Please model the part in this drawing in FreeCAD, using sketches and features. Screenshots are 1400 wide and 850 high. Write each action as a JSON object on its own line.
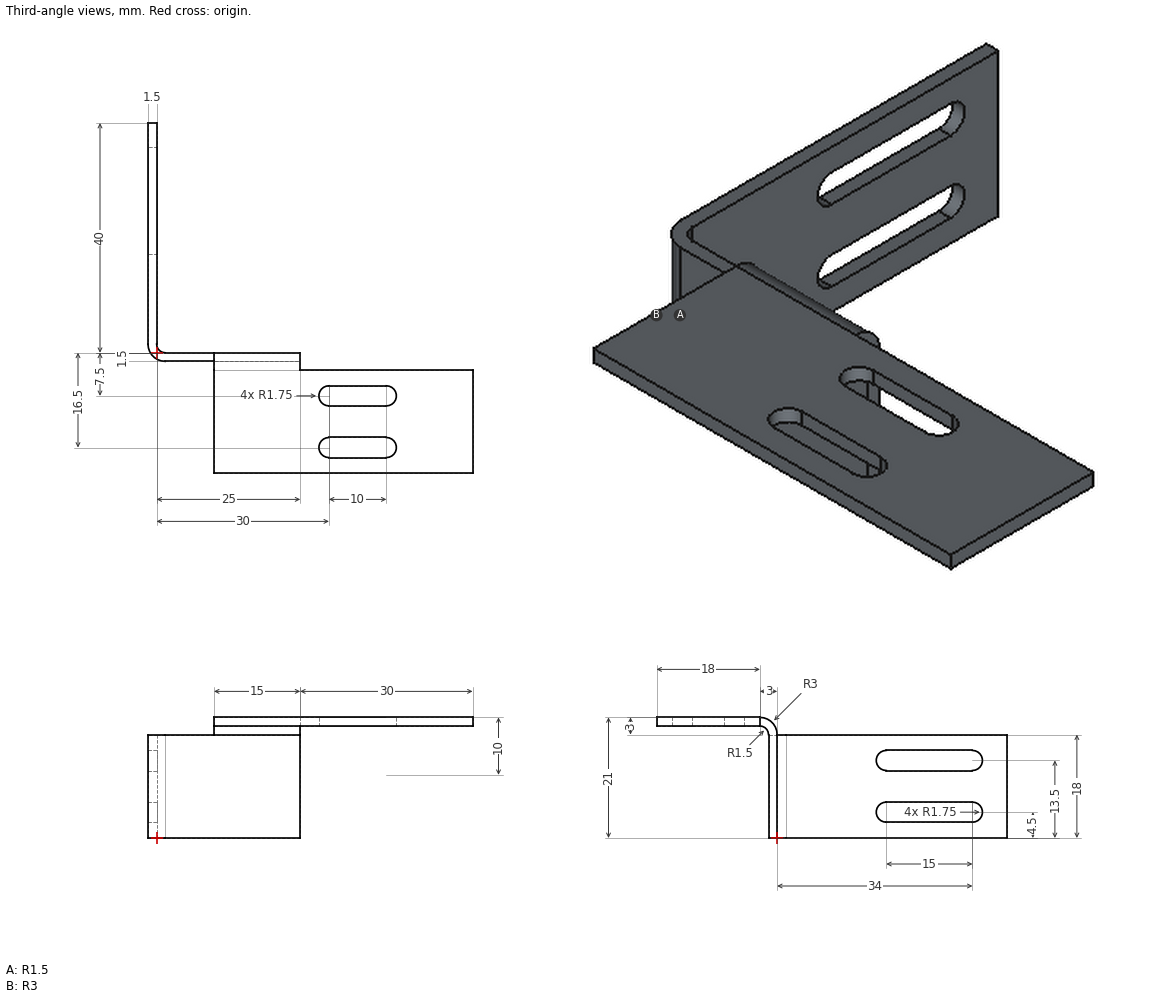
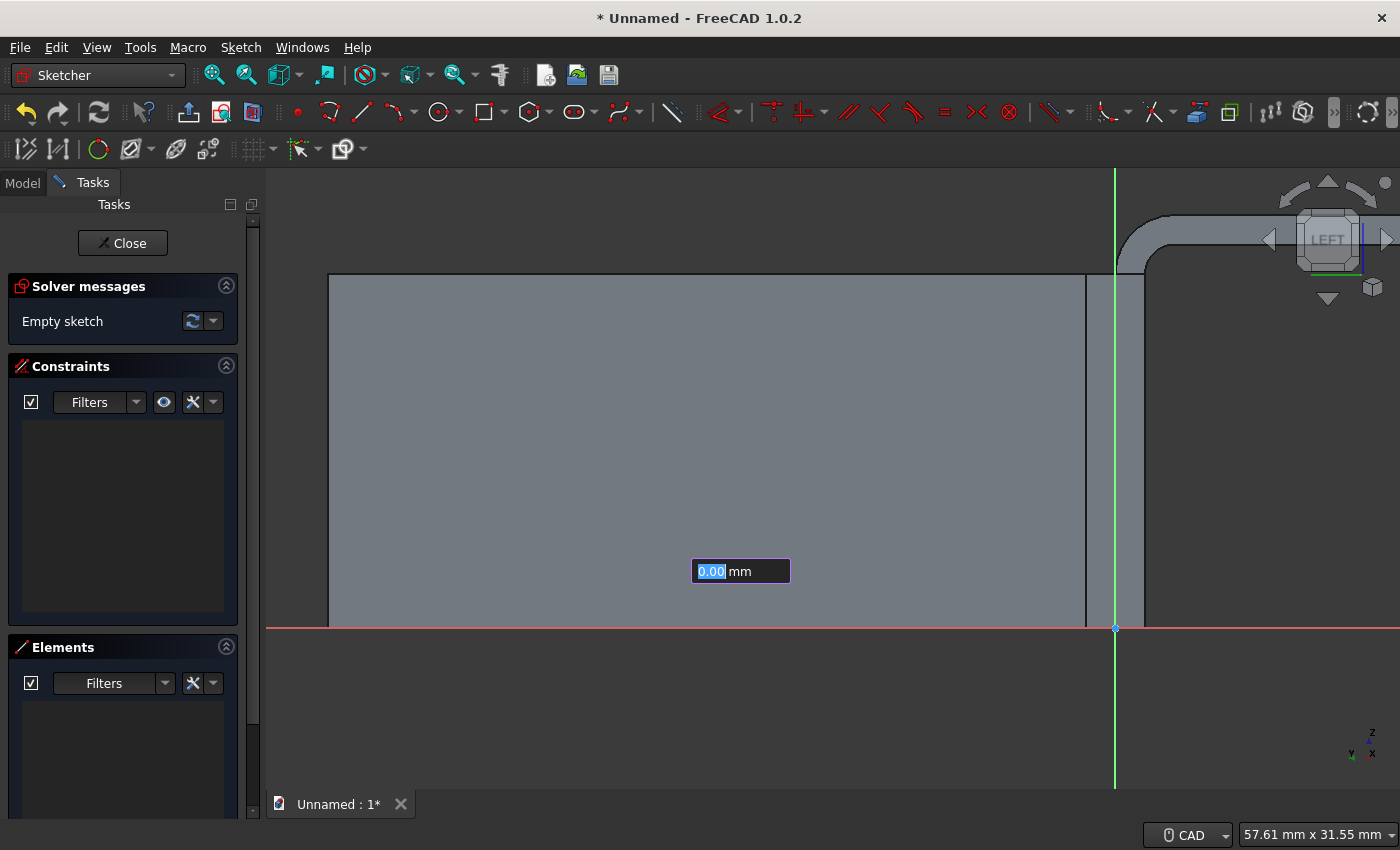
{"action": "left_click", "coordinate": [594, 505]}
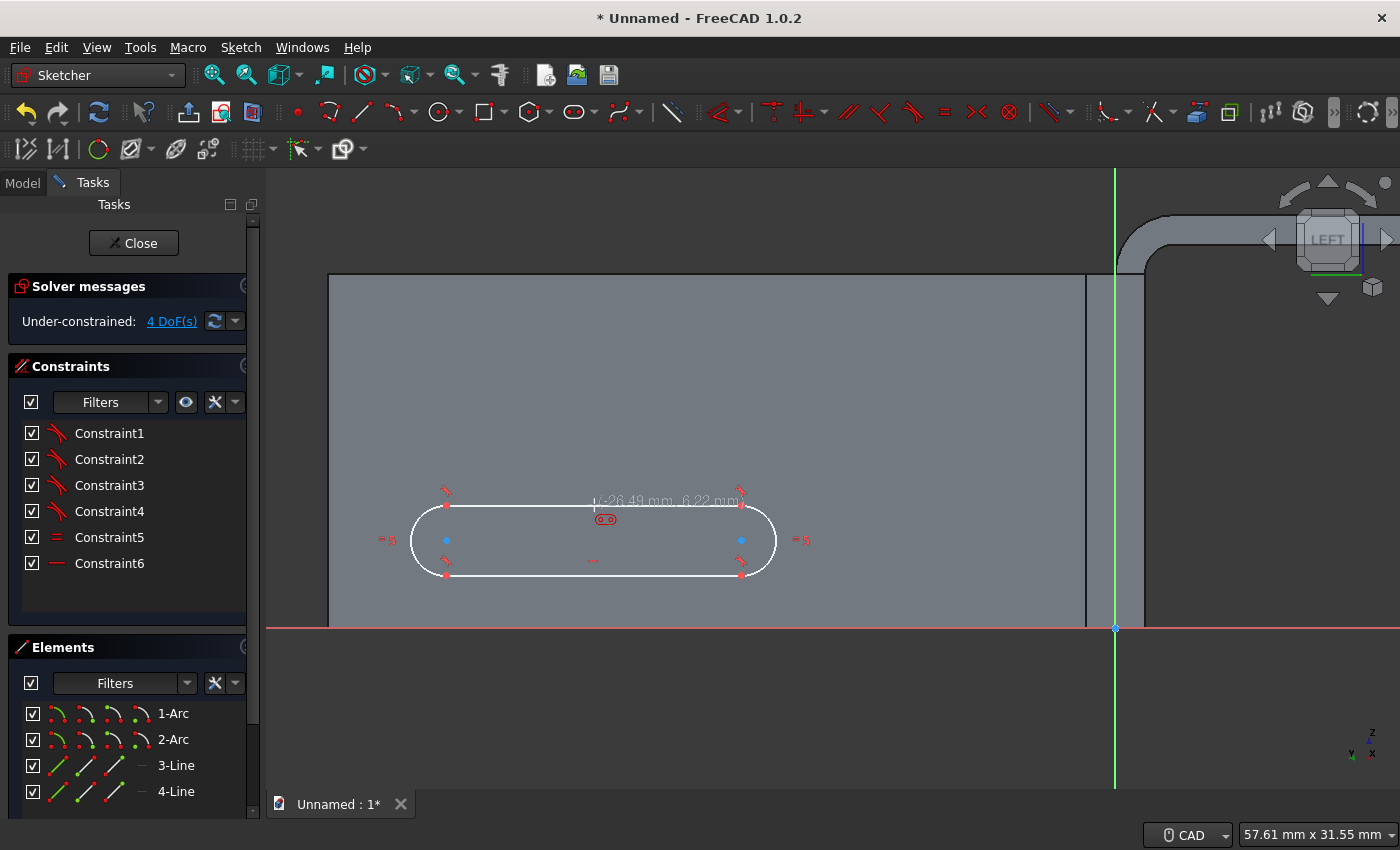
{"action": "left_click", "coordinate": [446, 363]}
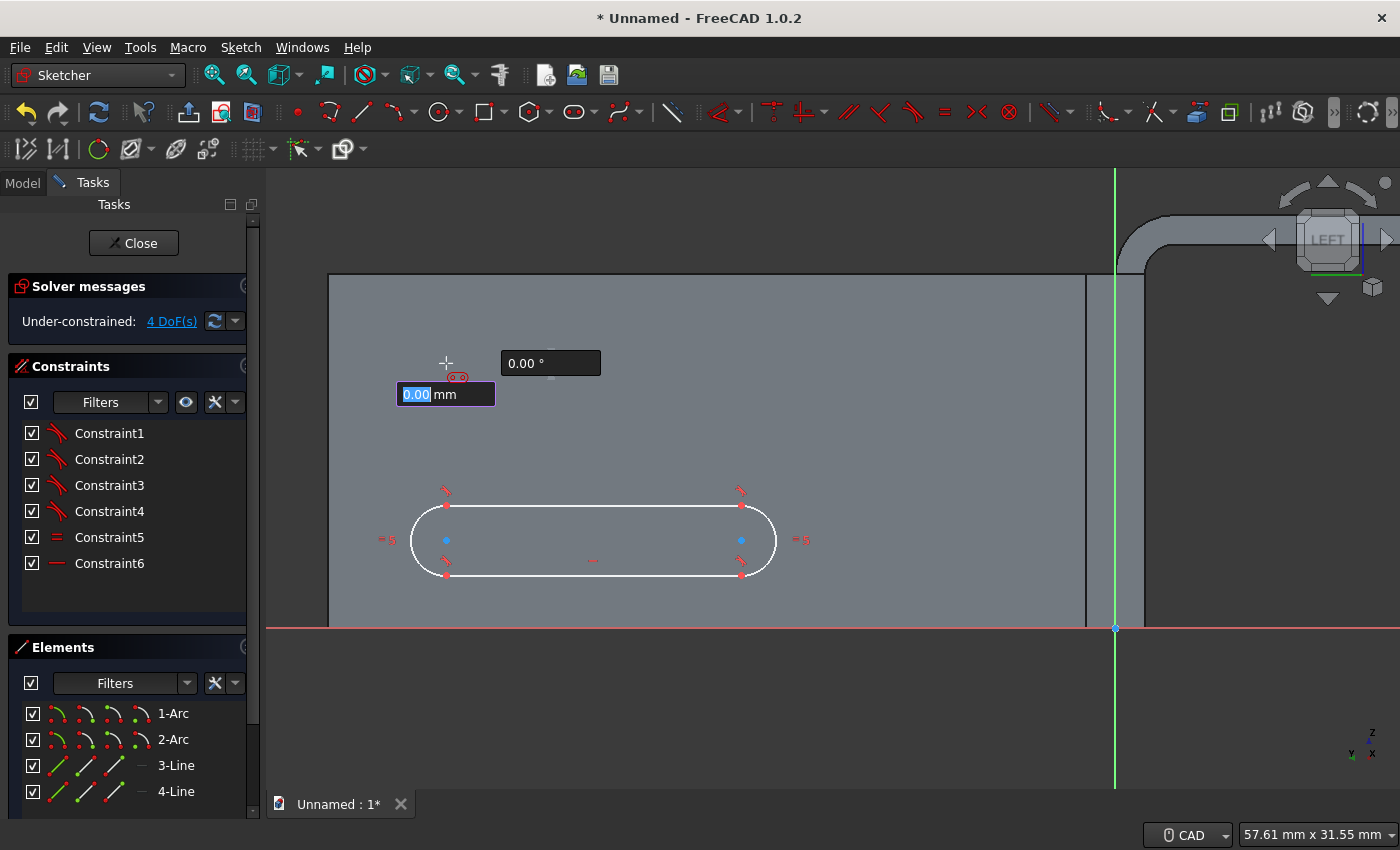
{"action": "left_click", "coordinate": [741, 363]}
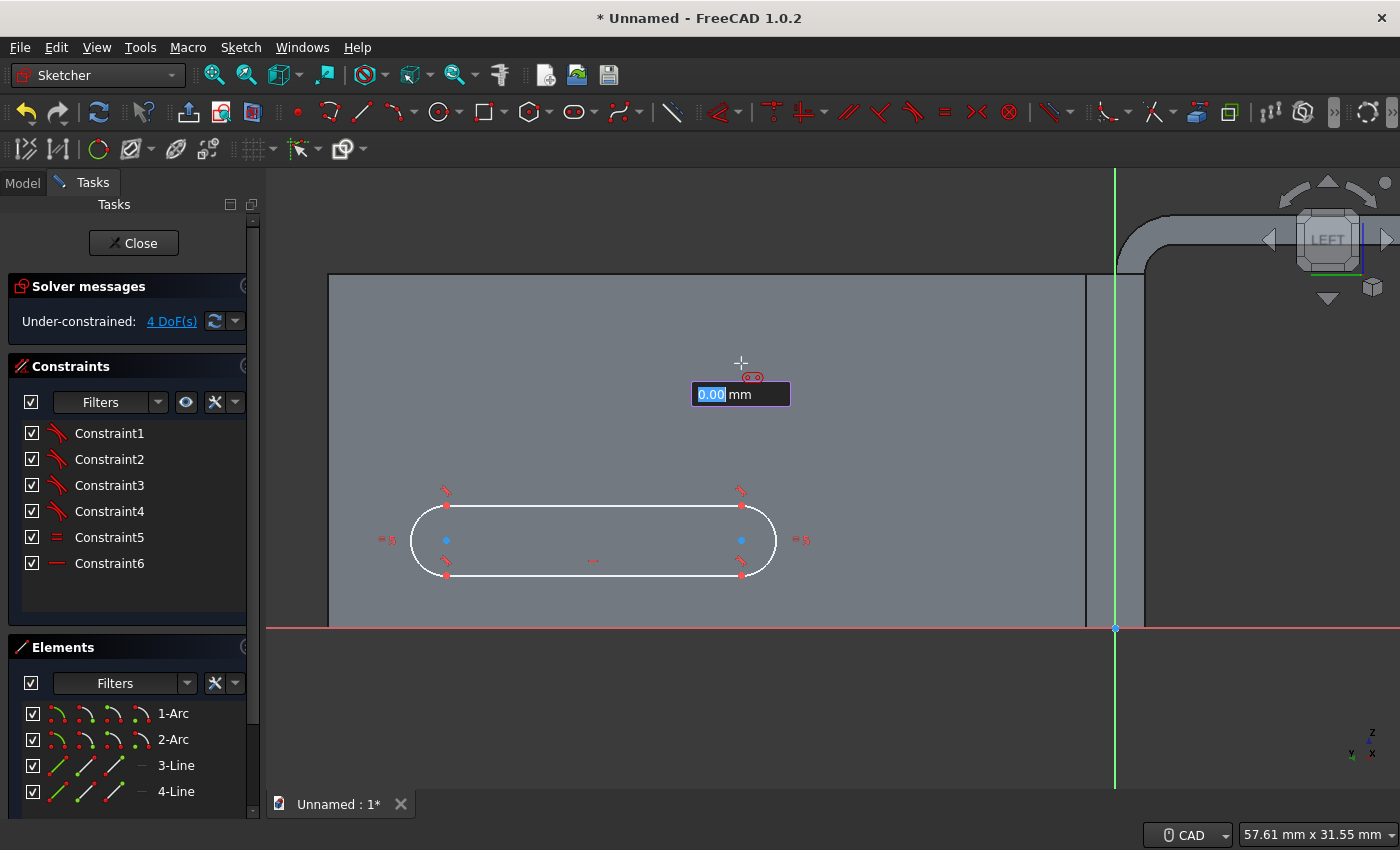
{"action": "left_click", "coordinate": [594, 397]}
{"action": "key", "text": "Escape"}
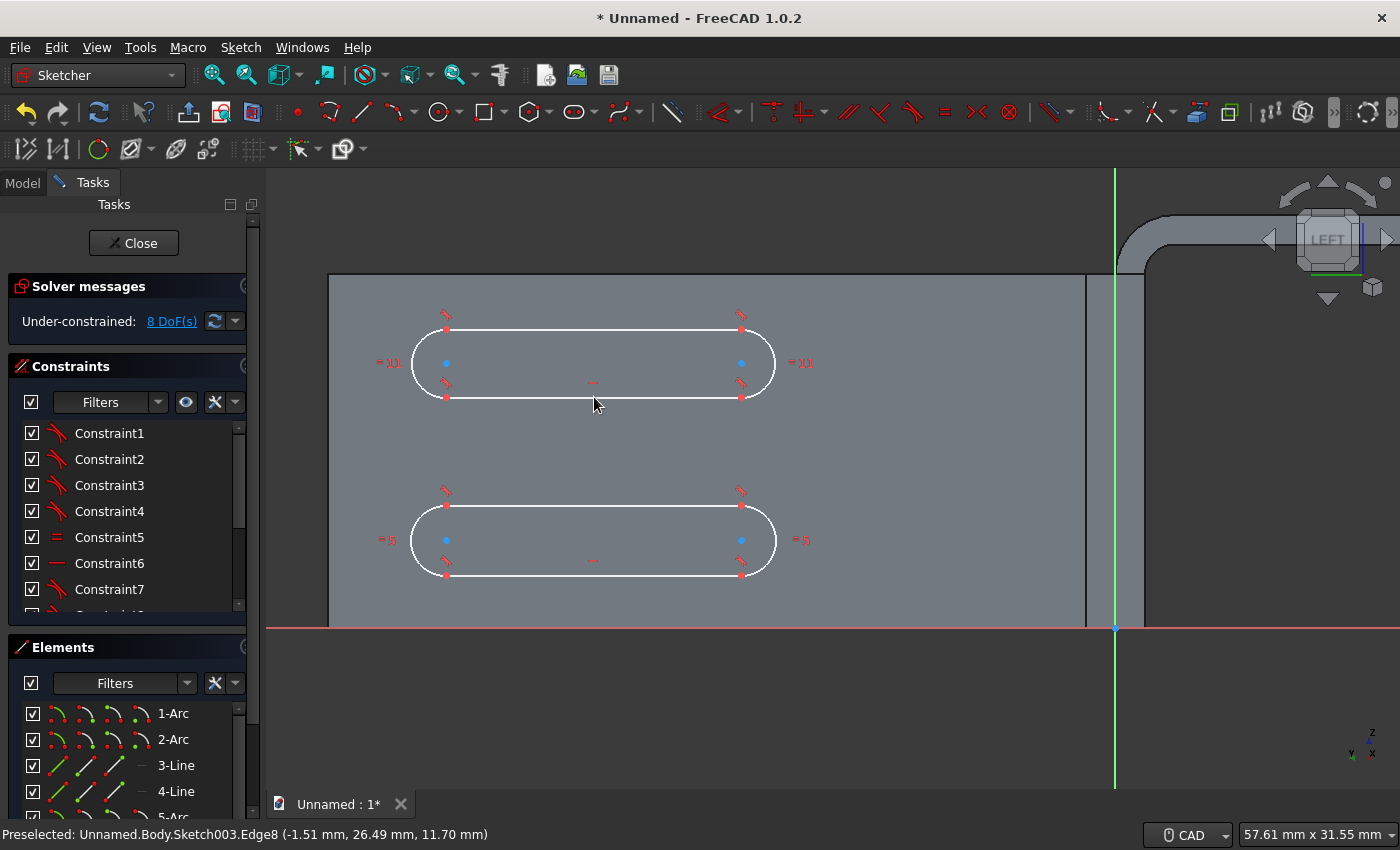
{"action": "left_click", "coordinate": [418, 520]}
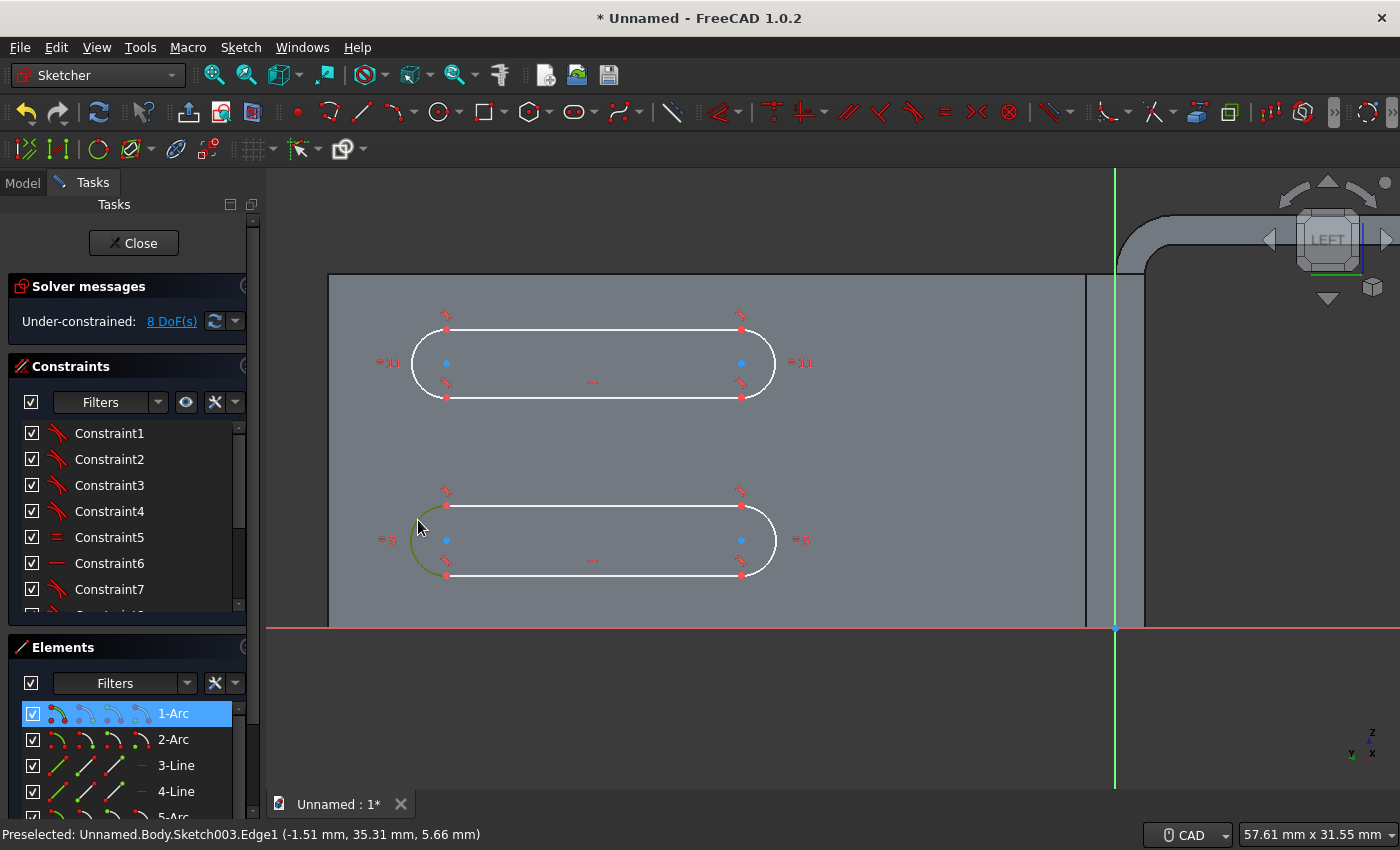
{"action": "left_click", "coordinate": [418, 344]}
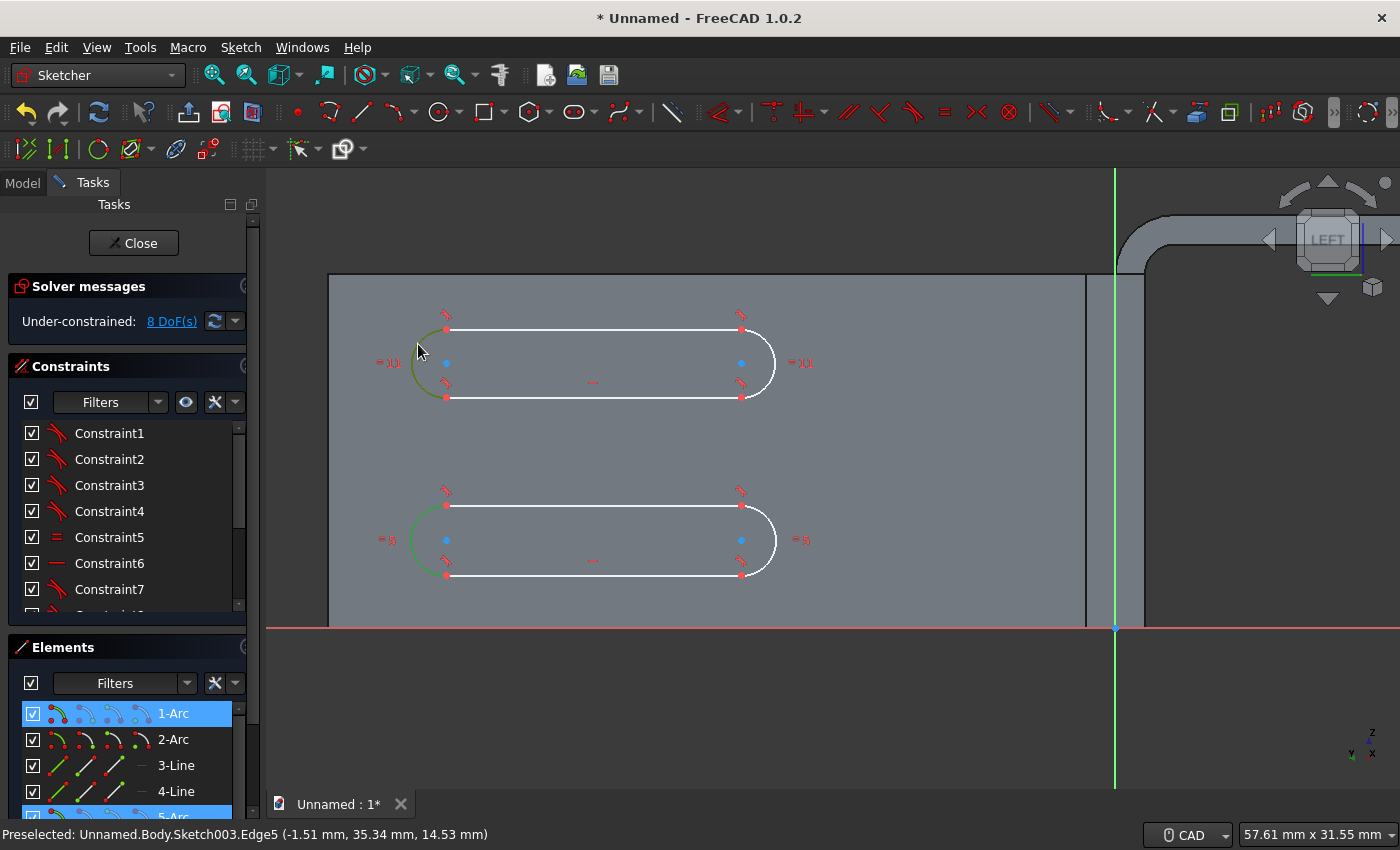
{"action": "key", "text": "e"}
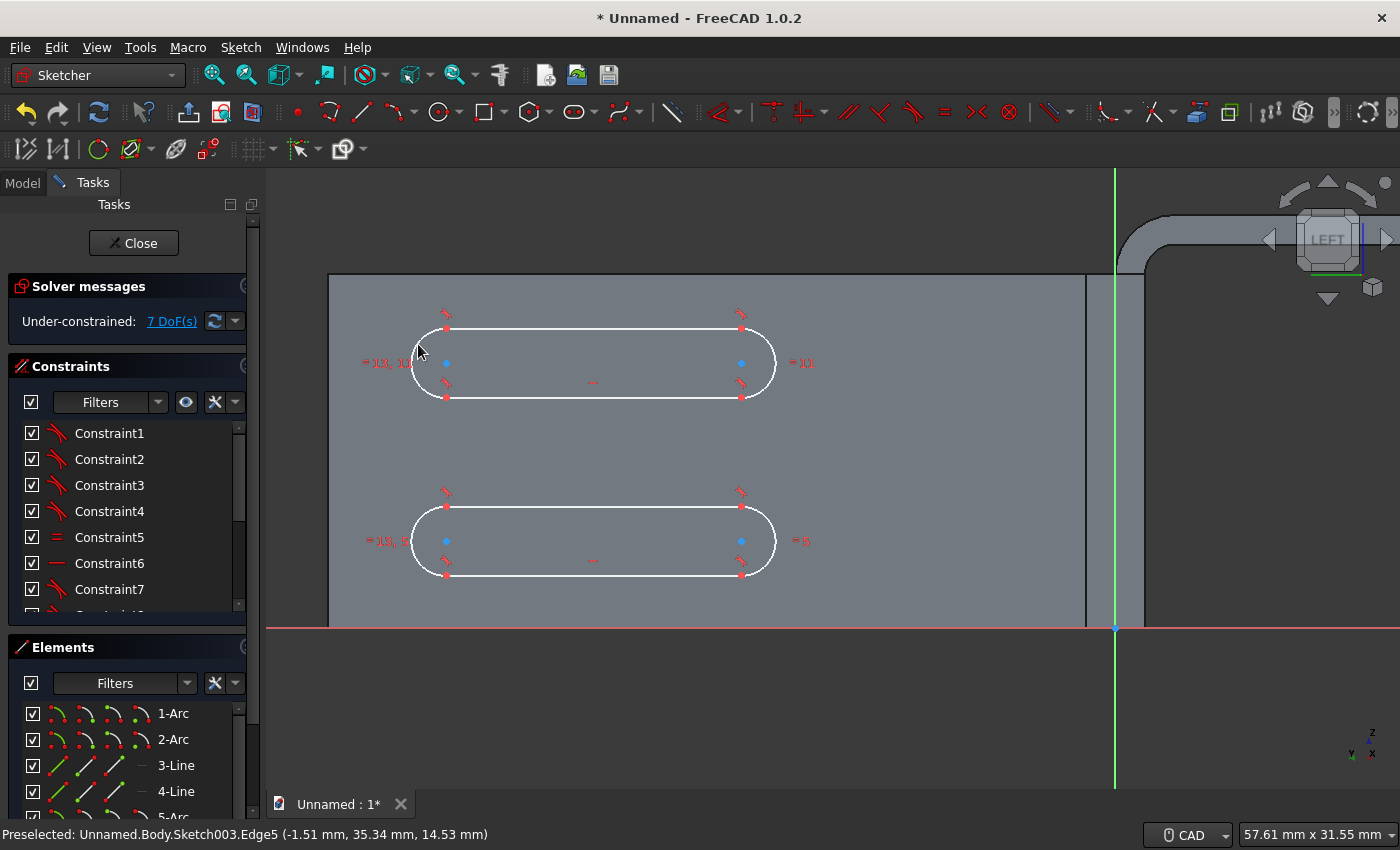
{"action": "key", "text": "d"}